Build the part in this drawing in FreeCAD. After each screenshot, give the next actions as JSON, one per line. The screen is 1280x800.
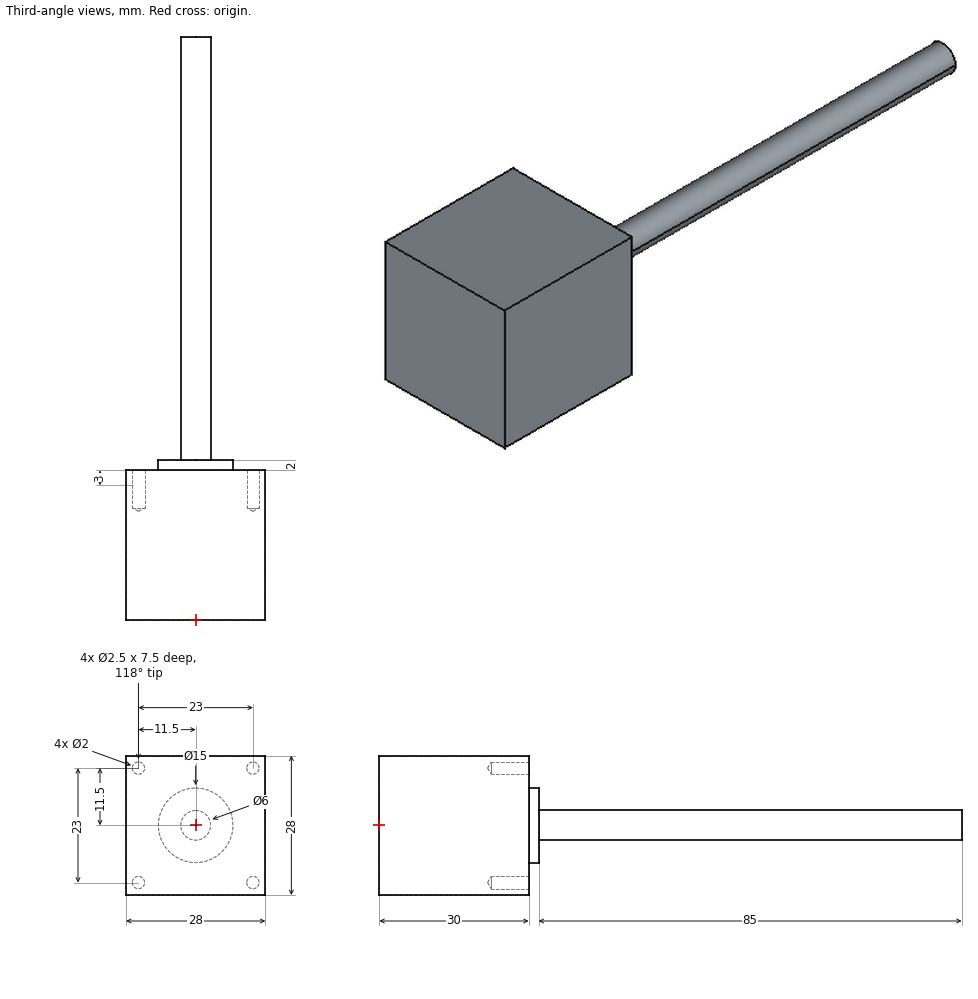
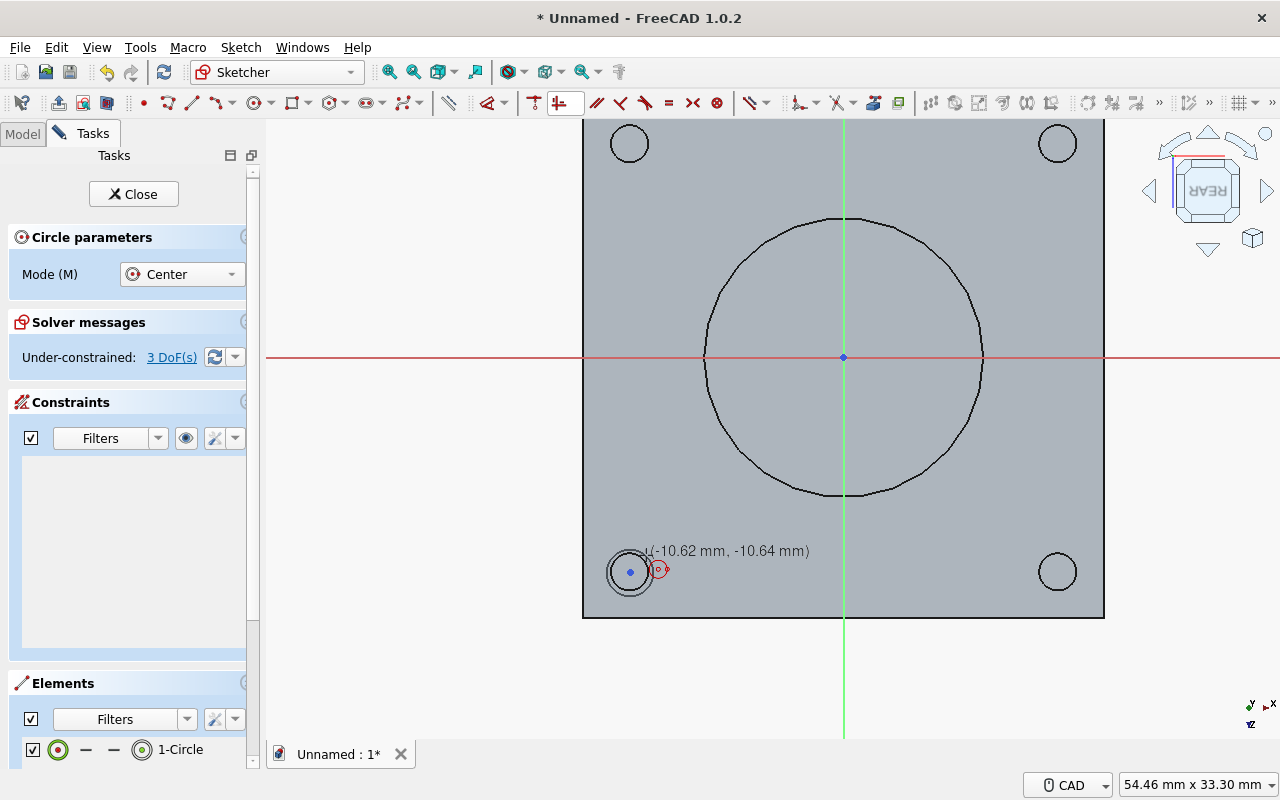
{"action": "left_click", "coordinate": [1058, 572]}
{"action": "left_click", "coordinate": [1074, 555]}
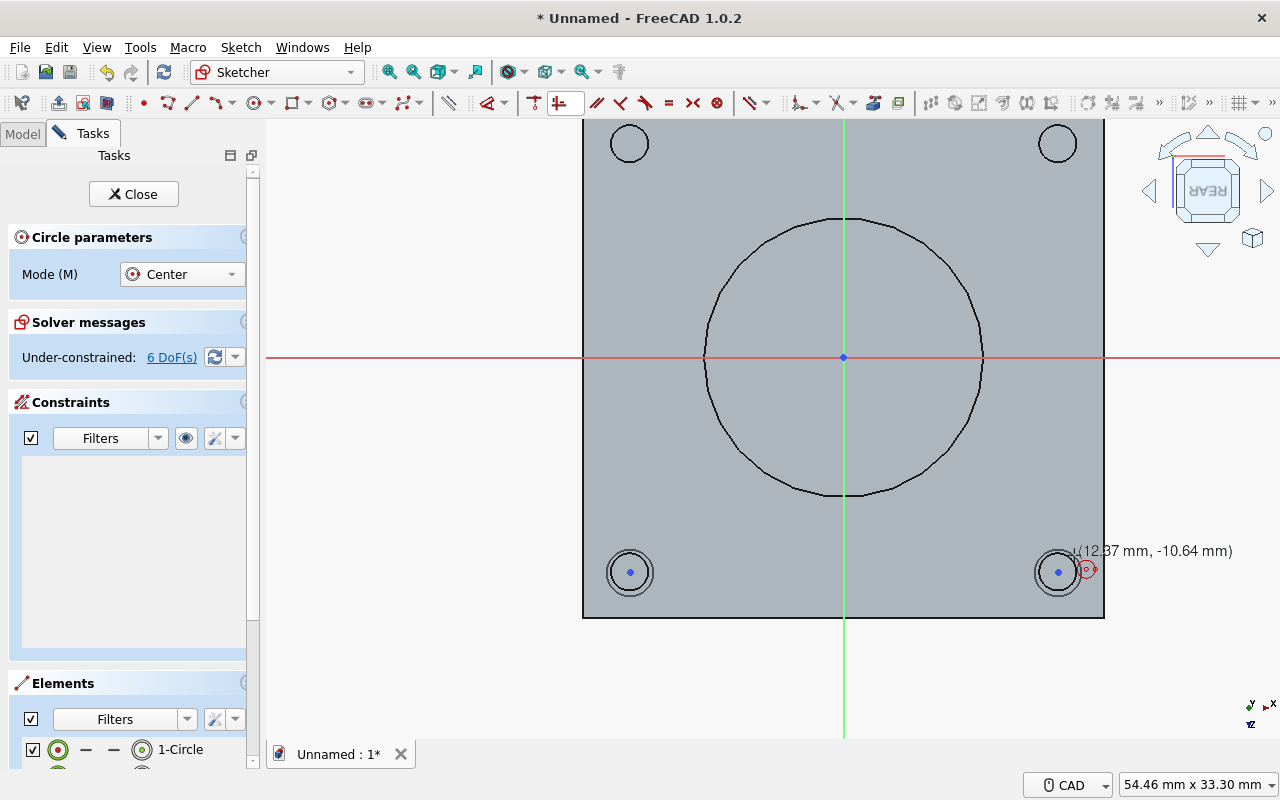
{"action": "scroll", "coordinate": [294, 711], "scroll_direction": "down", "scroll_amount": 1}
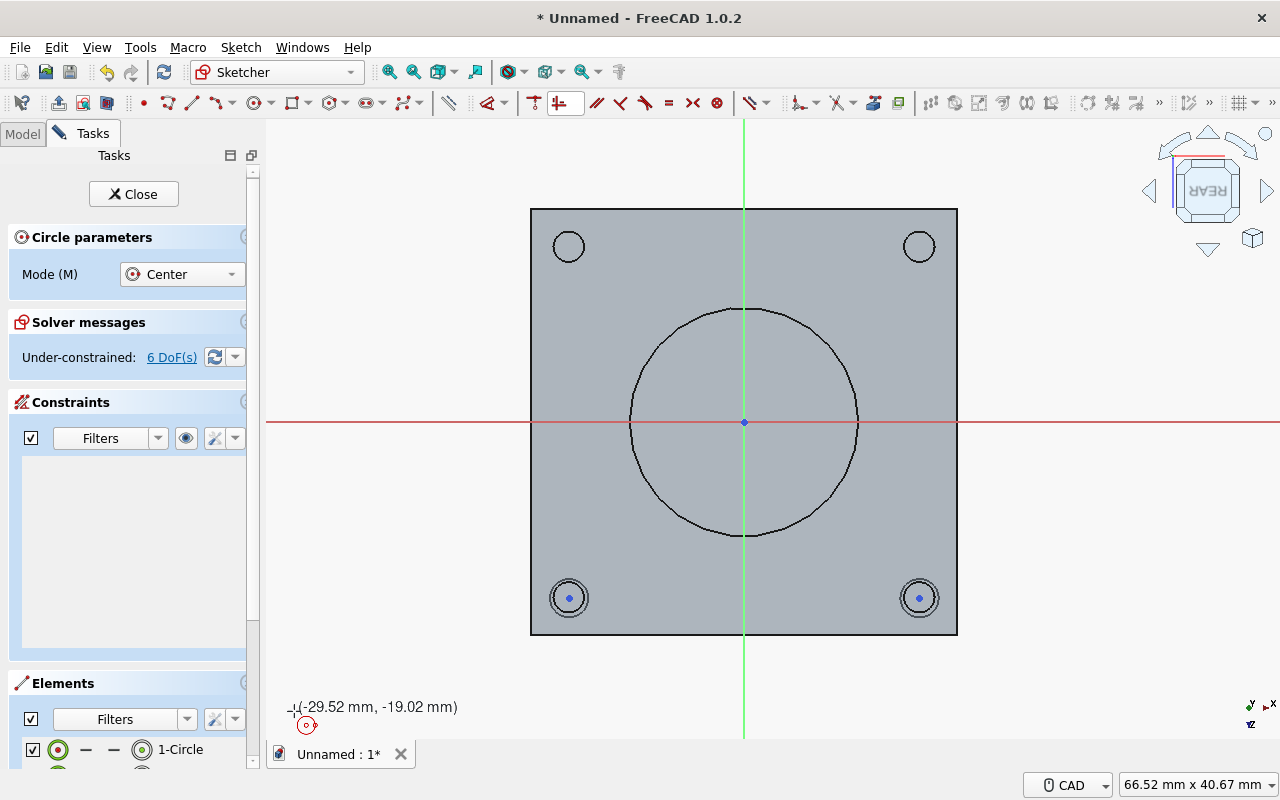
{"action": "left_click", "coordinate": [569, 247]}
{"action": "left_click", "coordinate": [582, 233]}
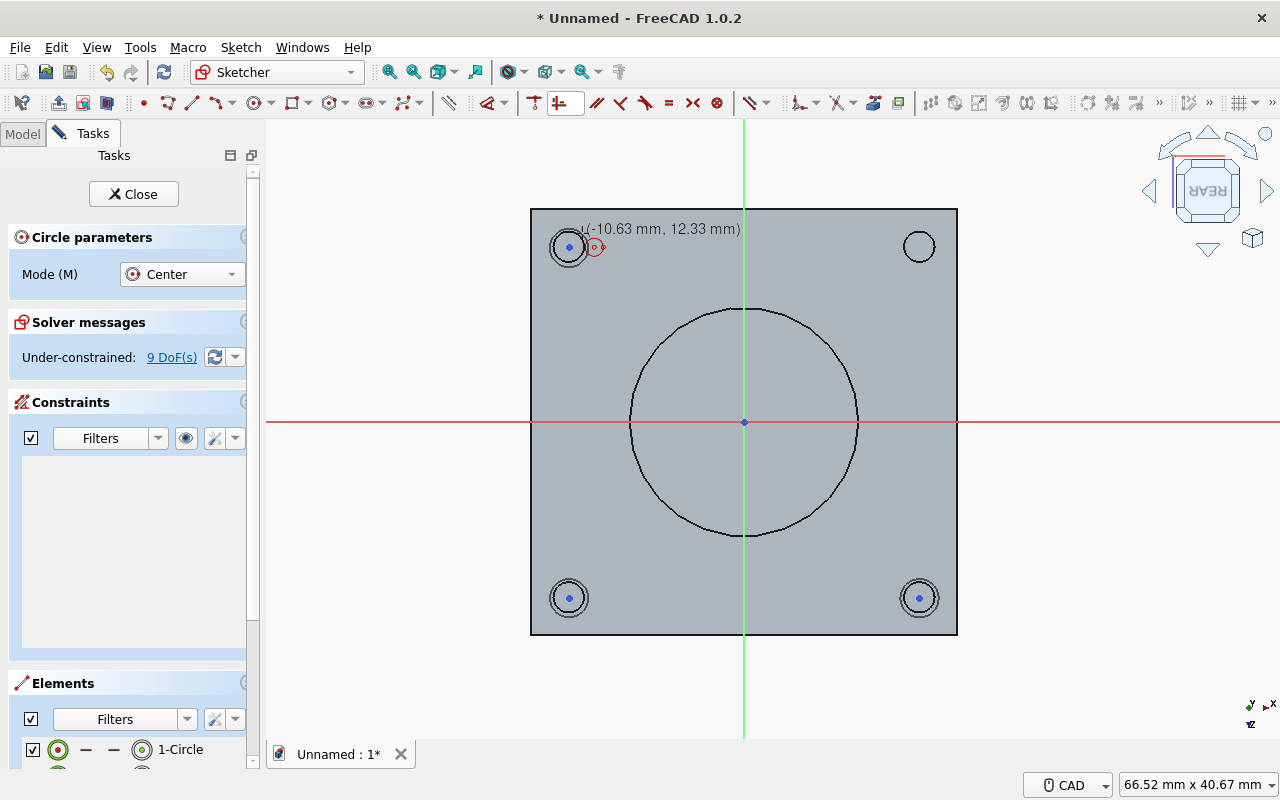
{"action": "left_click", "coordinate": [919, 247]}
{"action": "left_click", "coordinate": [933, 233]}
{"action": "key", "text": "Escape"}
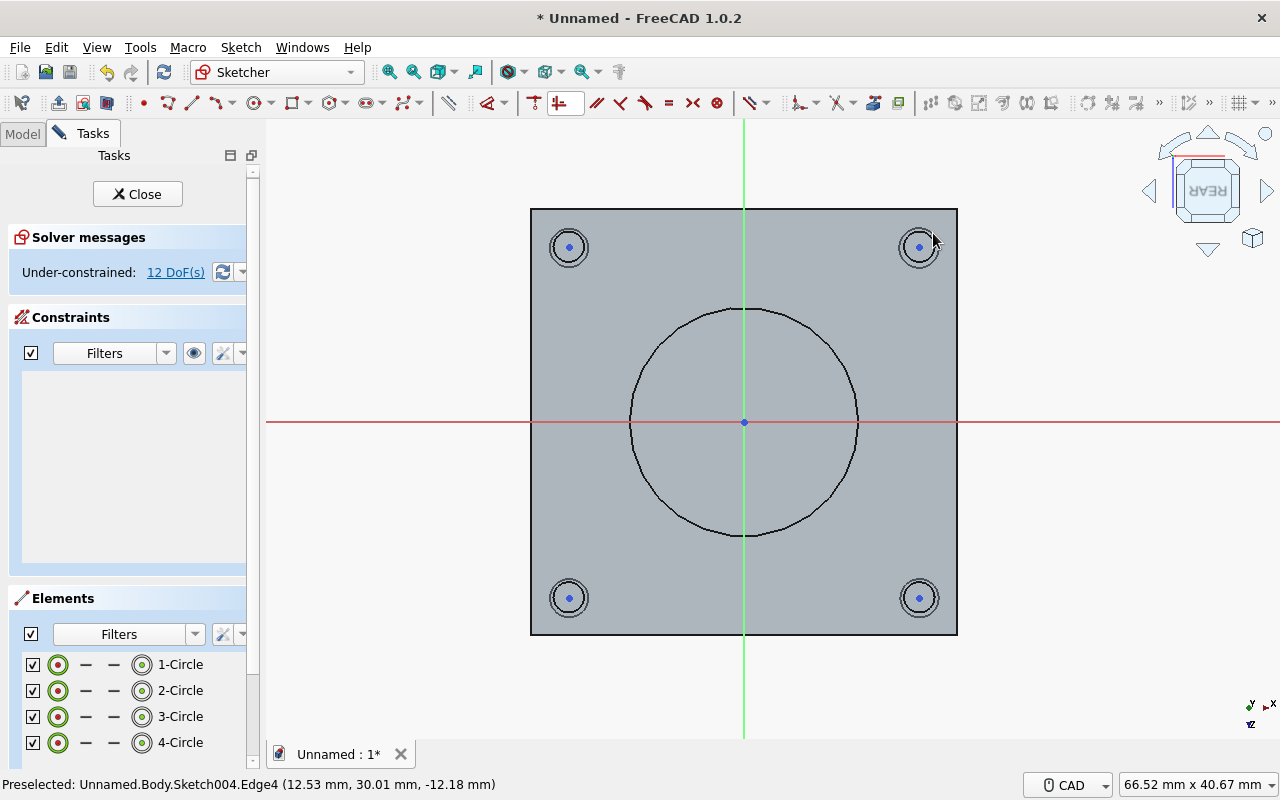
{"action": "left_click", "coordinate": [583, 585]}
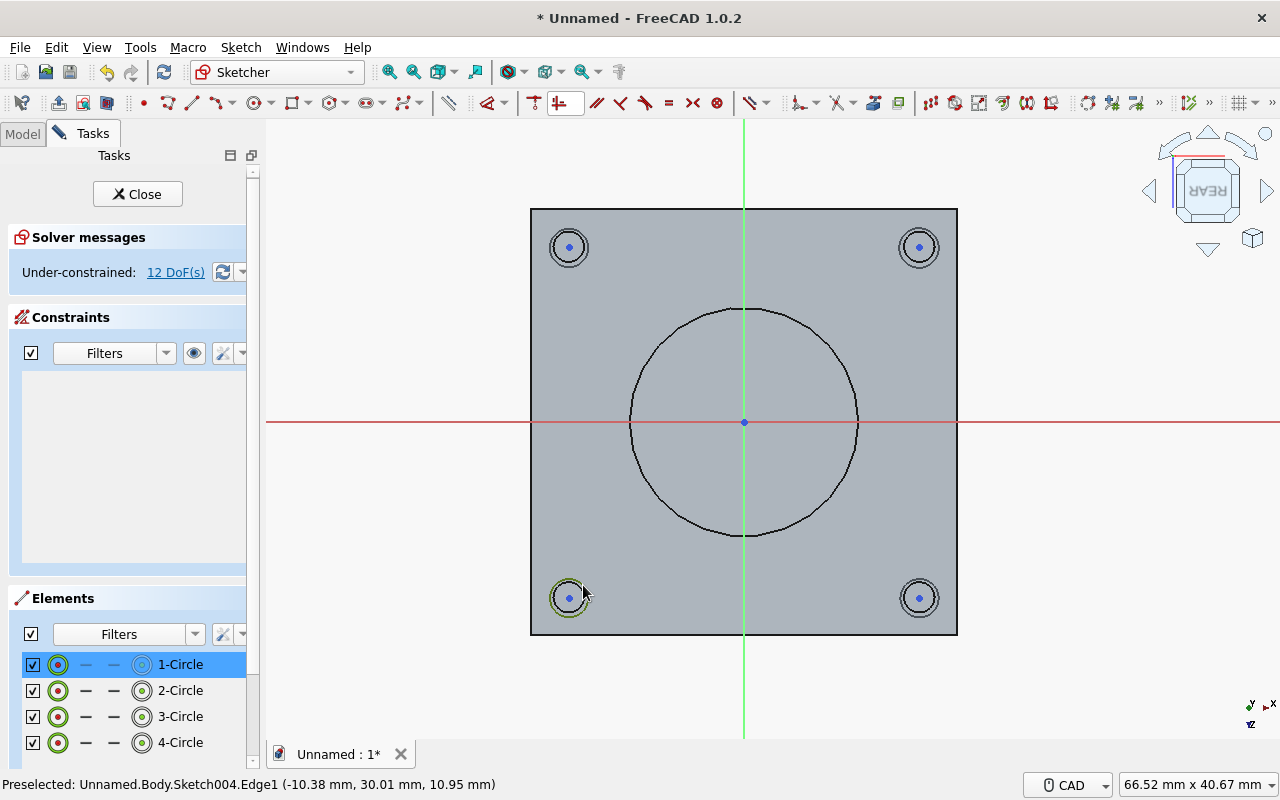
{"action": "left_click", "coordinate": [933, 585]}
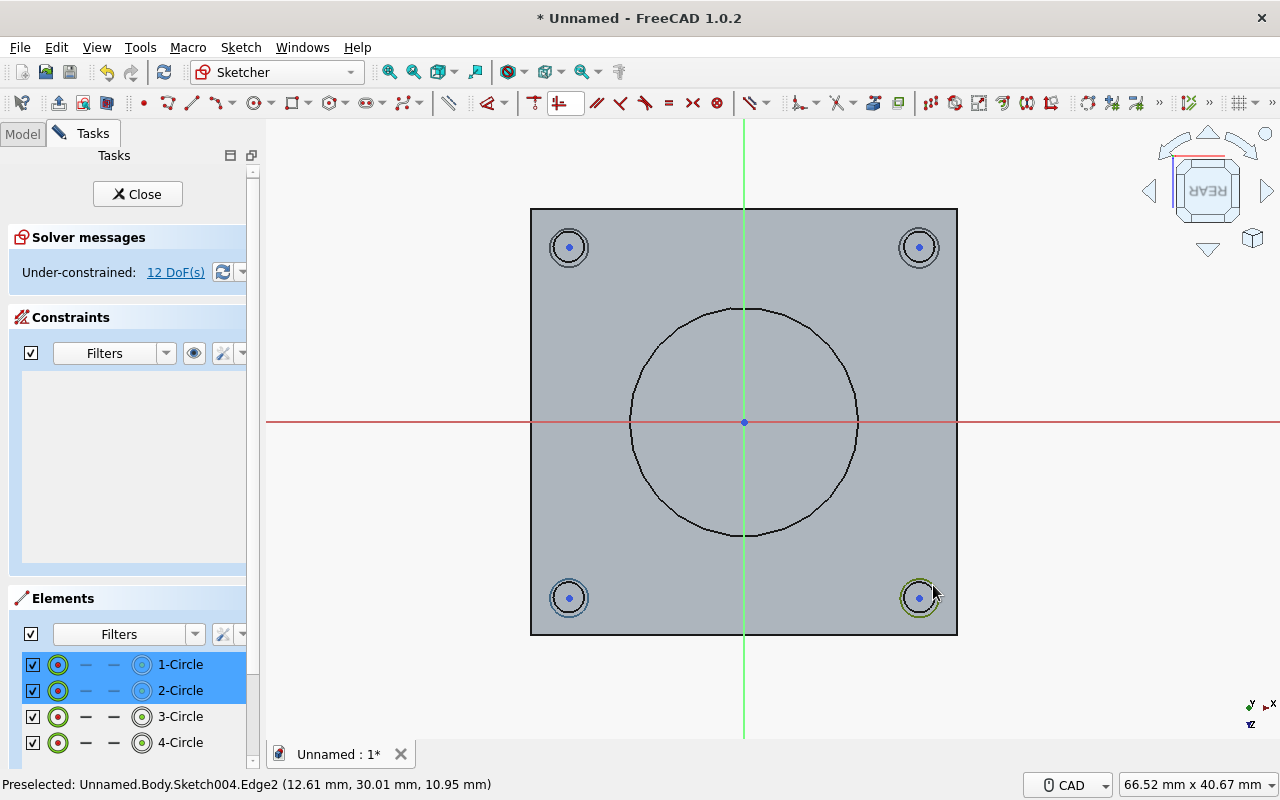
{"action": "left_click", "coordinate": [582, 234]}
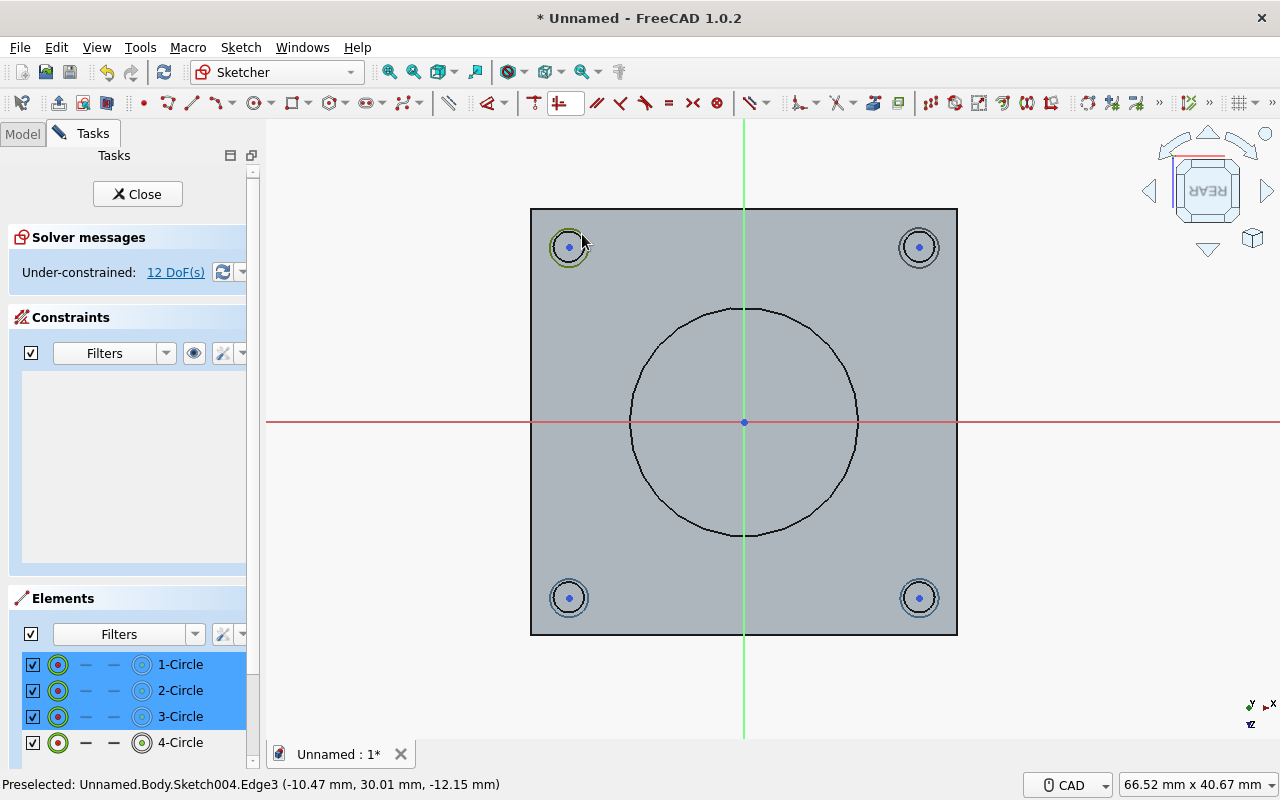
{"action": "left_click", "coordinate": [933, 234]}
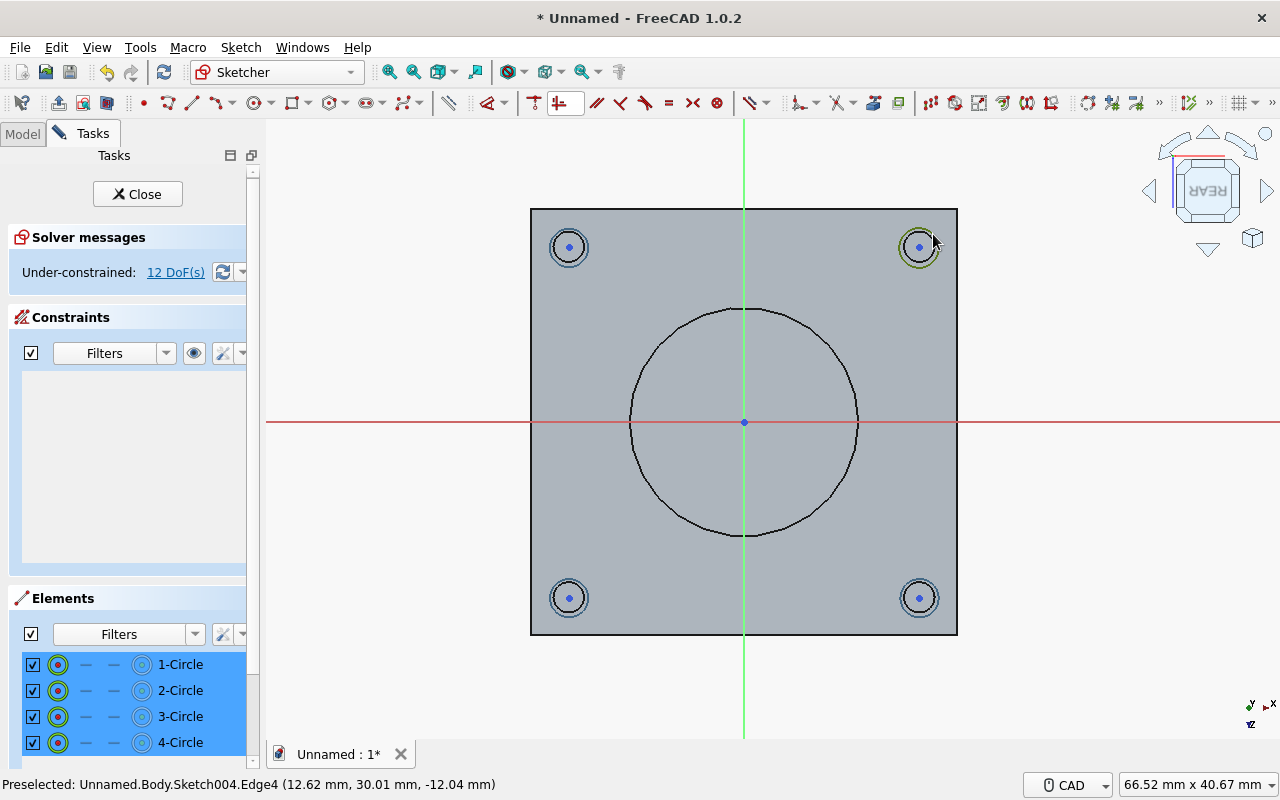
{"action": "left_click", "coordinate": [670, 104]}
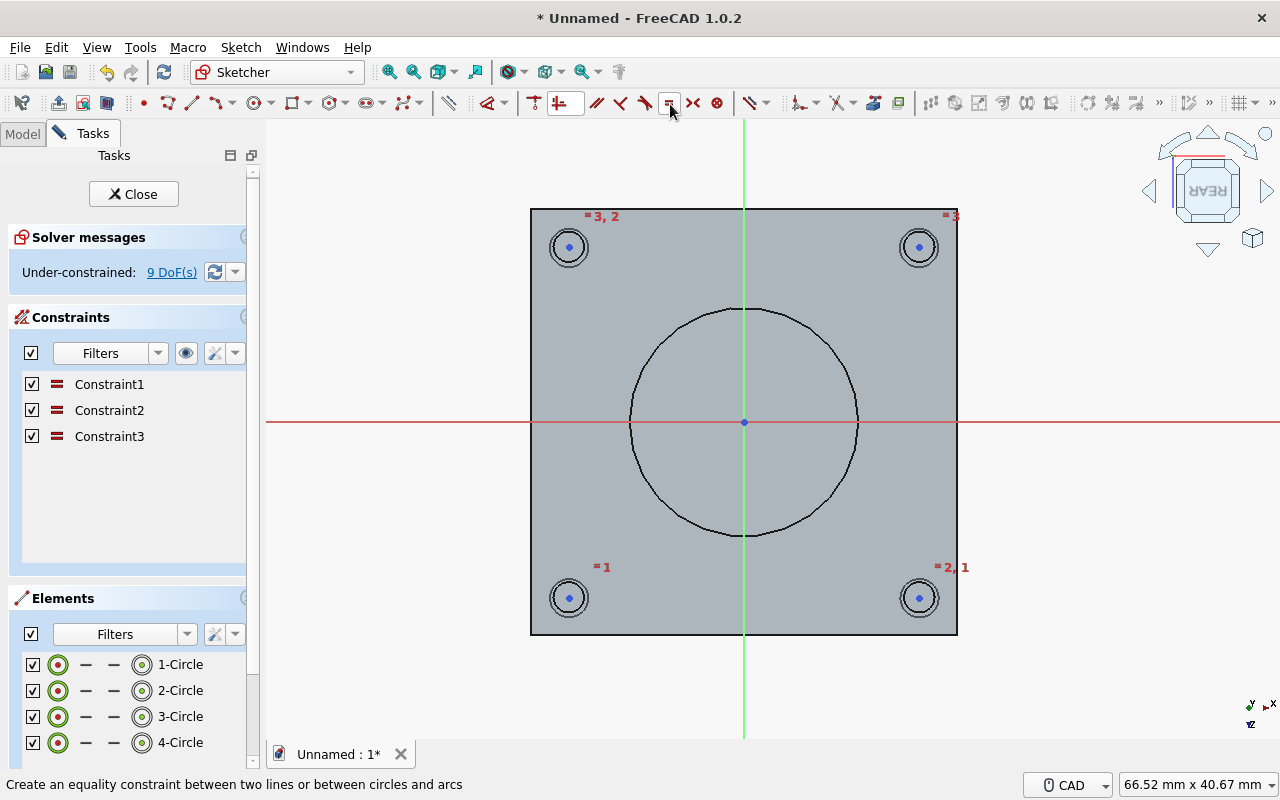
{"action": "left_click", "coordinate": [569, 598]}